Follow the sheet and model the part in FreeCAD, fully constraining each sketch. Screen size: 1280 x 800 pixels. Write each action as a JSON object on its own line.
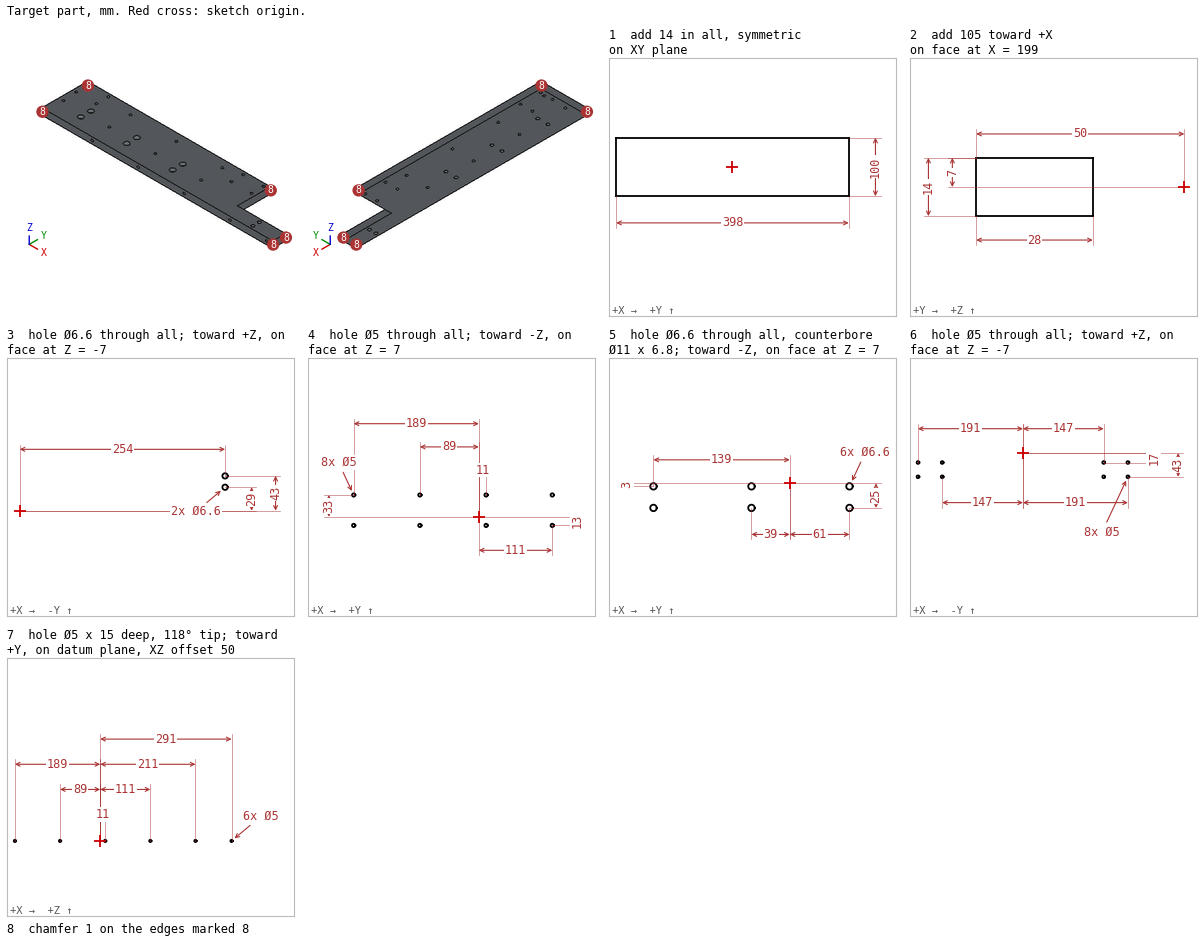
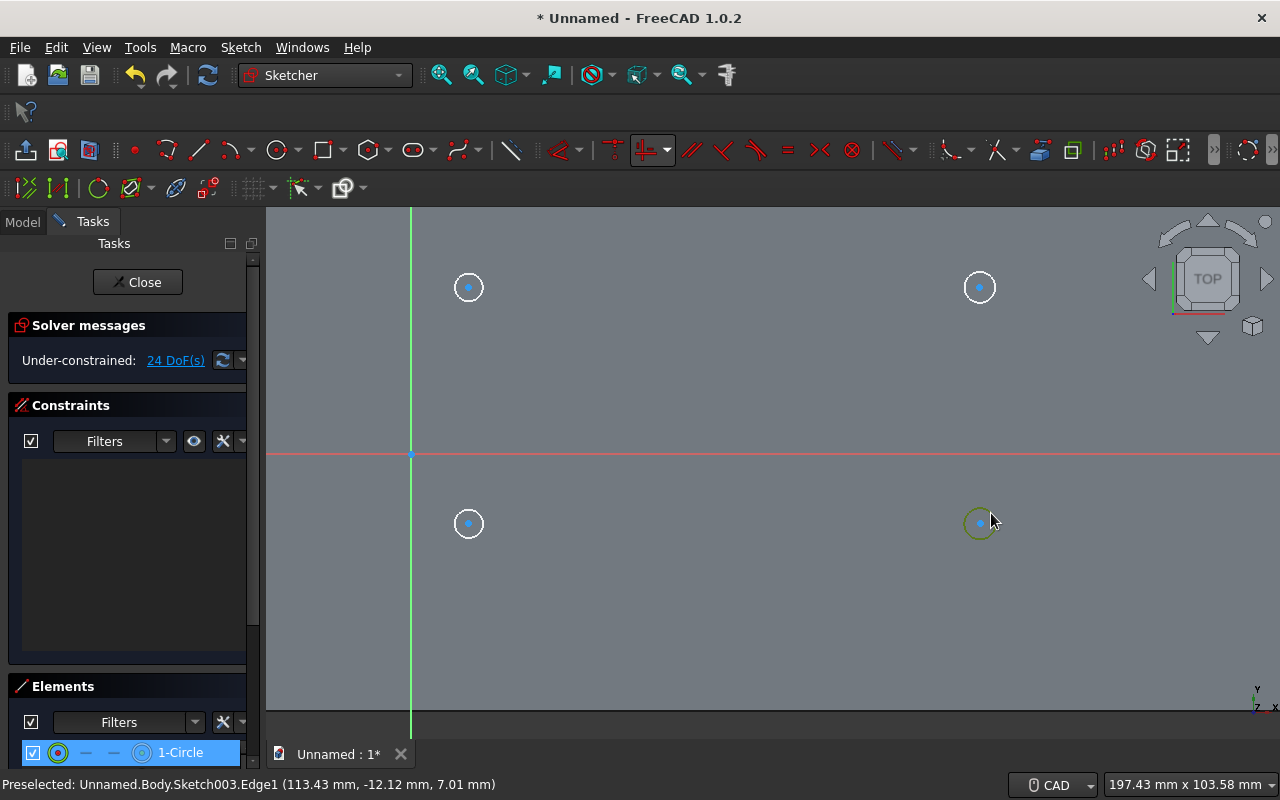
{"action": "scroll", "coordinate": [992, 514], "scroll_direction": "down", "scroll_amount": 5}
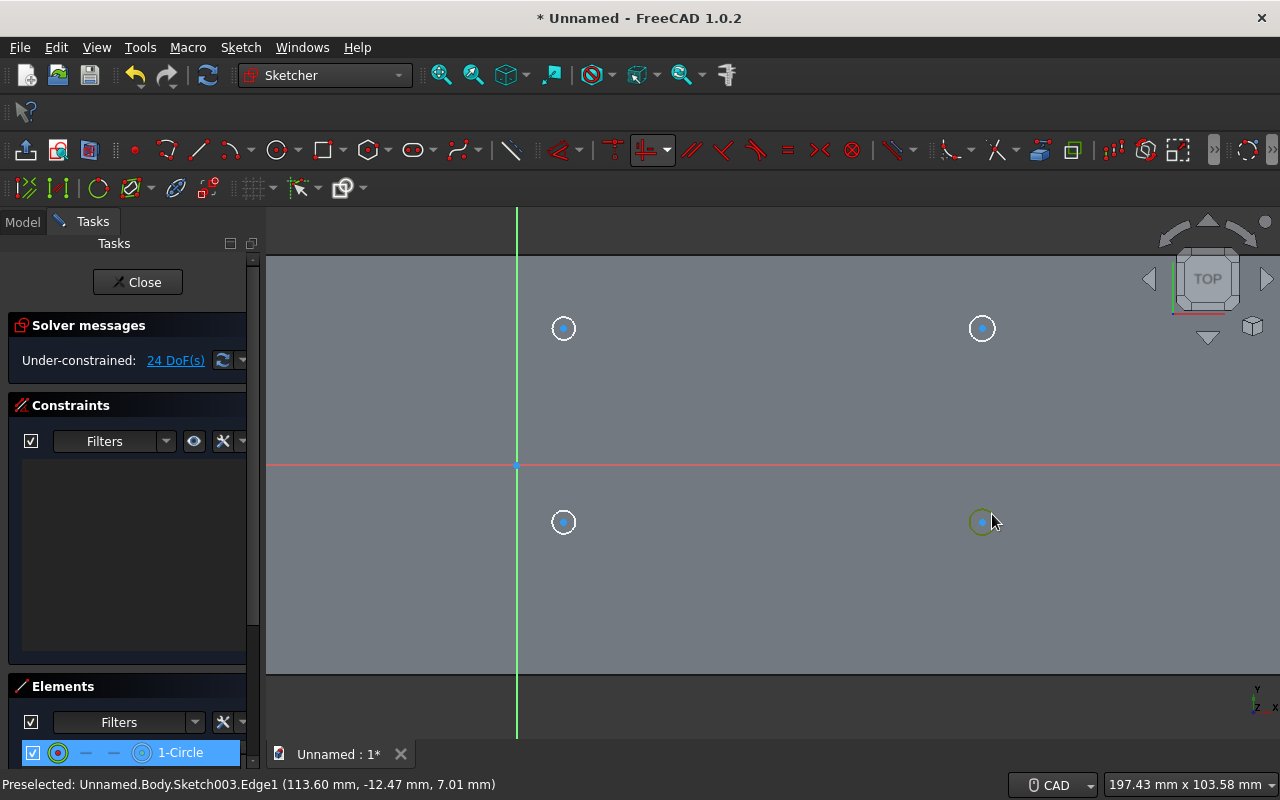
{"action": "scroll", "coordinate": [426, 427], "scroll_direction": "up", "scroll_amount": 6}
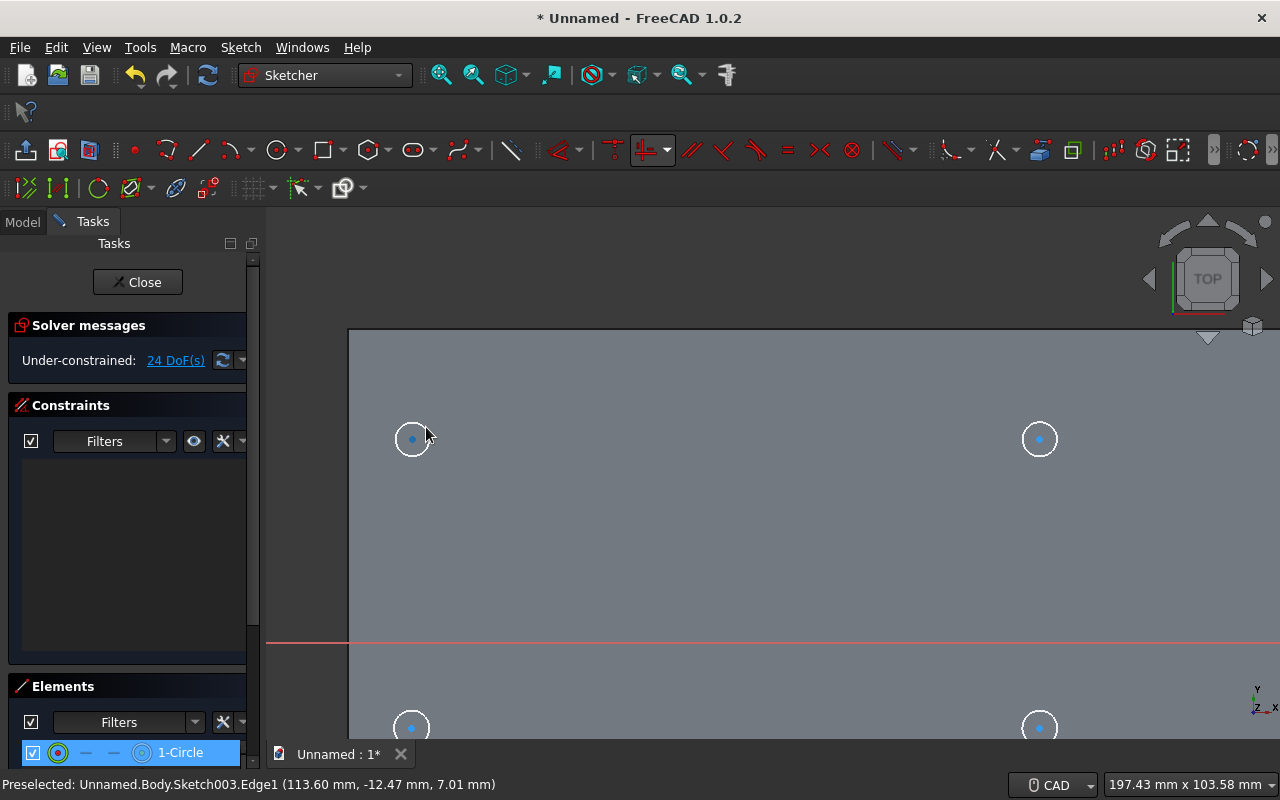
{"action": "left_click", "coordinate": [424, 427]}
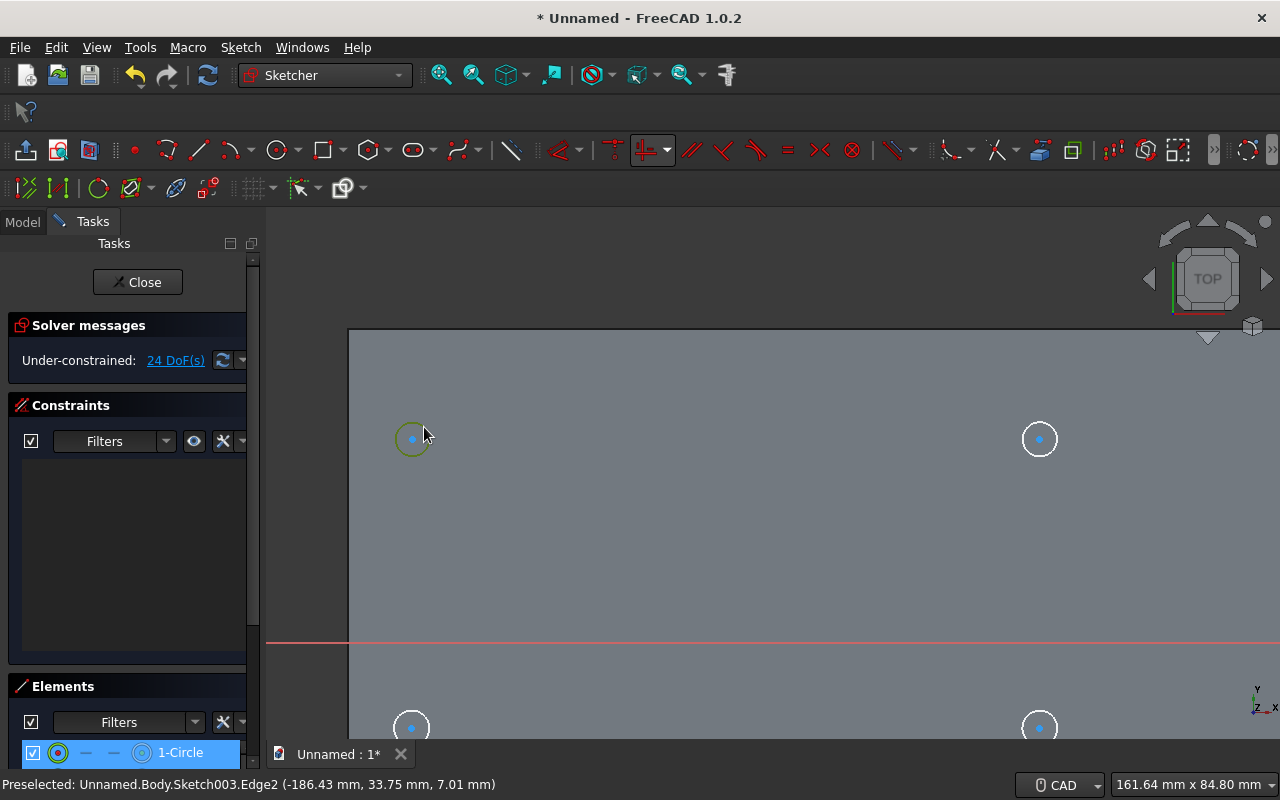
{"action": "left_click", "coordinate": [412, 711]}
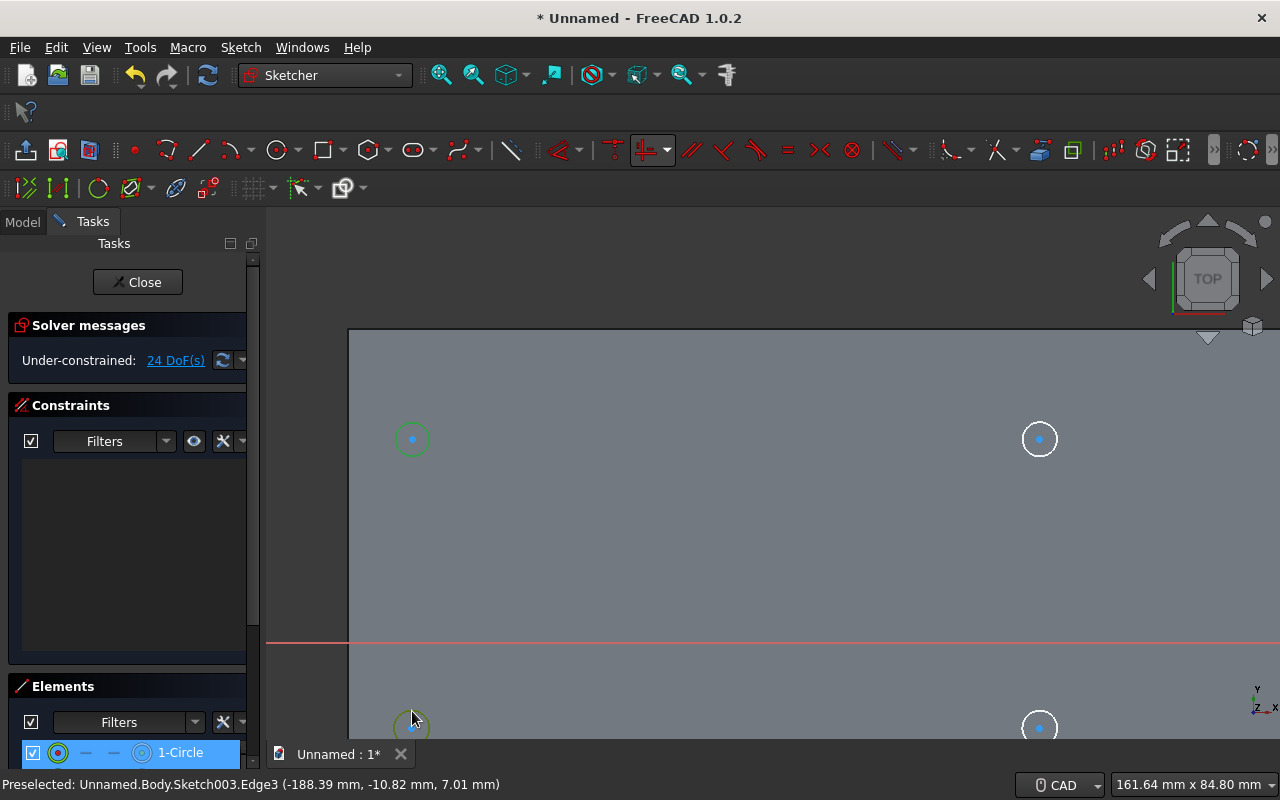
{"action": "left_click", "coordinate": [1052, 427]}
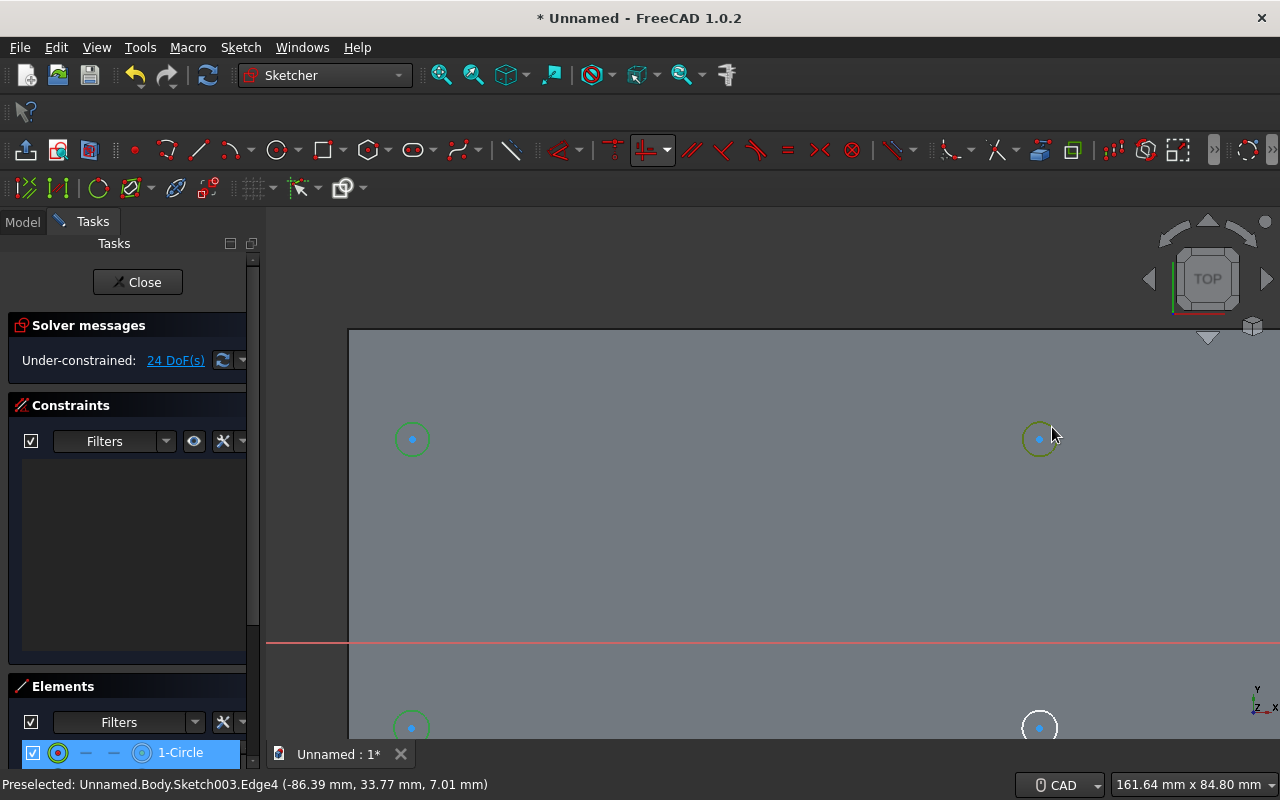
{"action": "left_click", "coordinate": [1040, 711]}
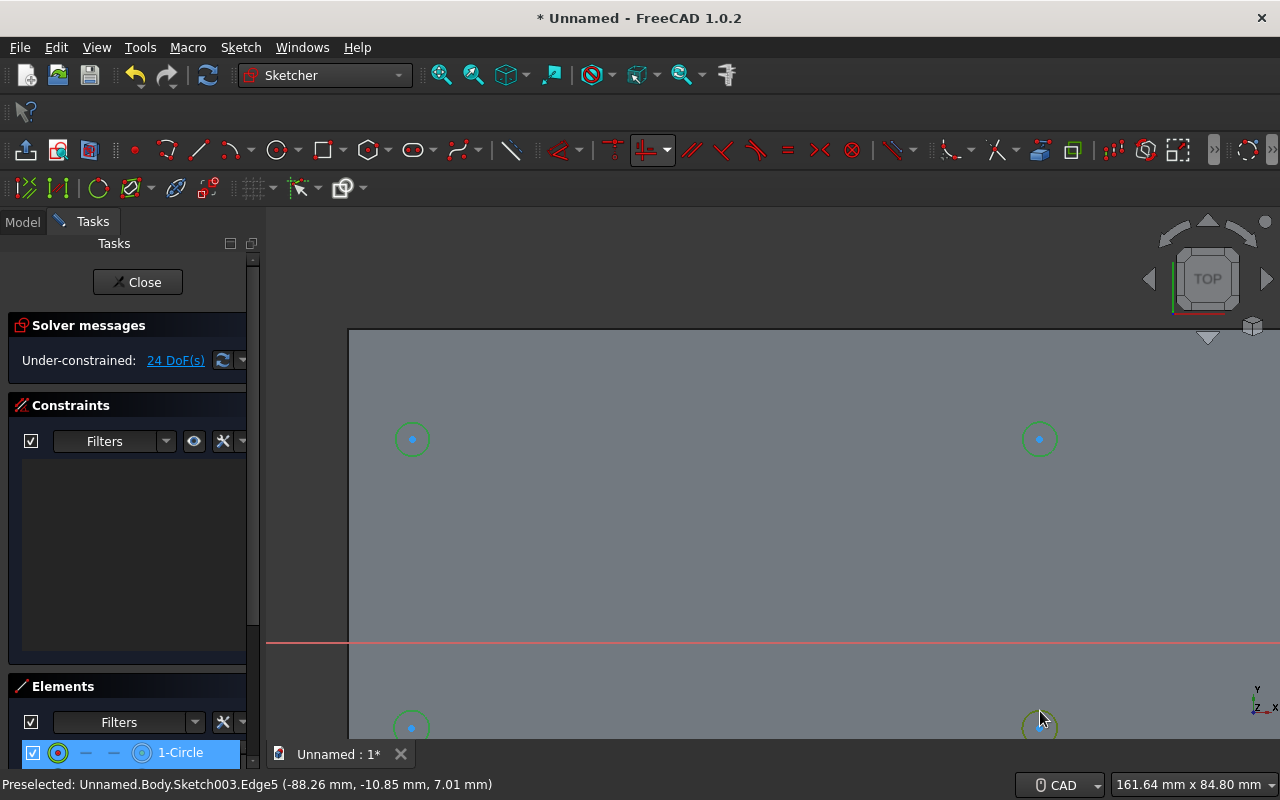
{"action": "scroll", "coordinate": [425, 427], "scroll_direction": "down", "scroll_amount": 6}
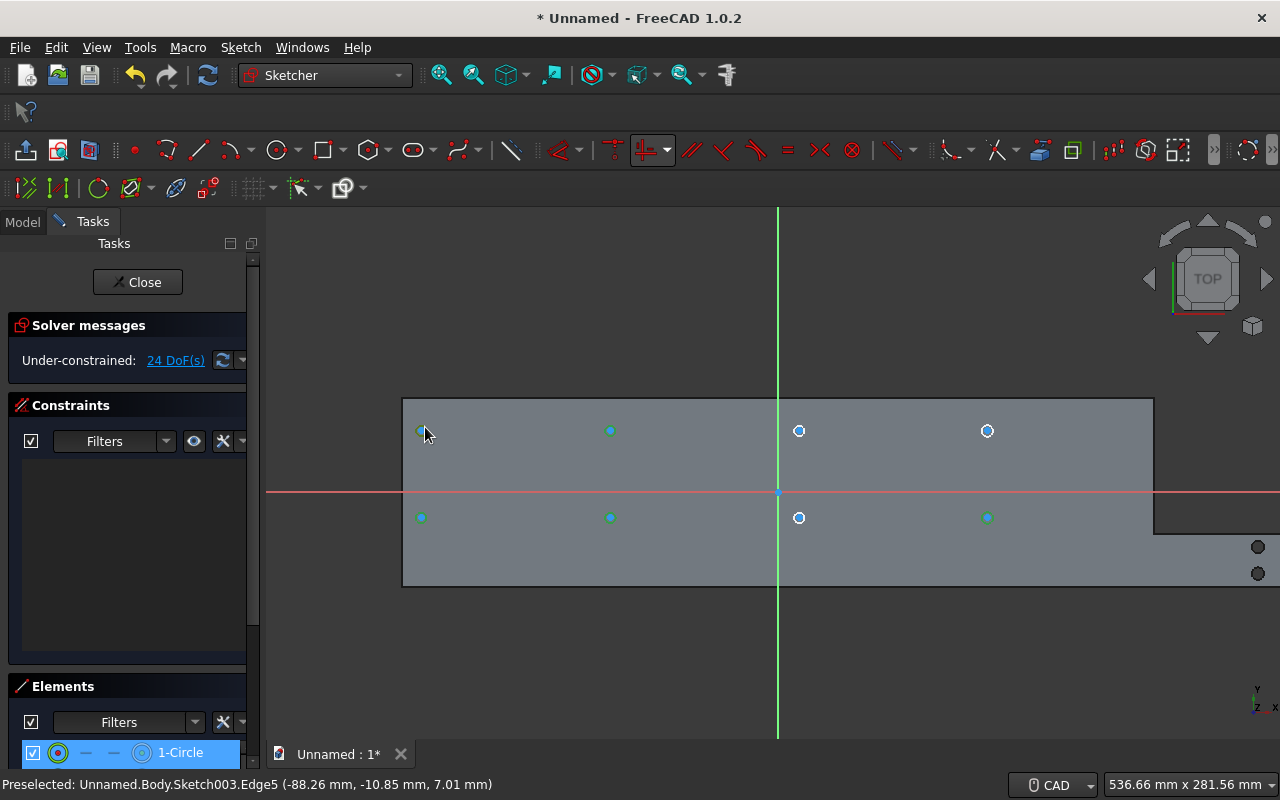
{"action": "scroll", "coordinate": [803, 427], "scroll_direction": "up", "scroll_amount": 5}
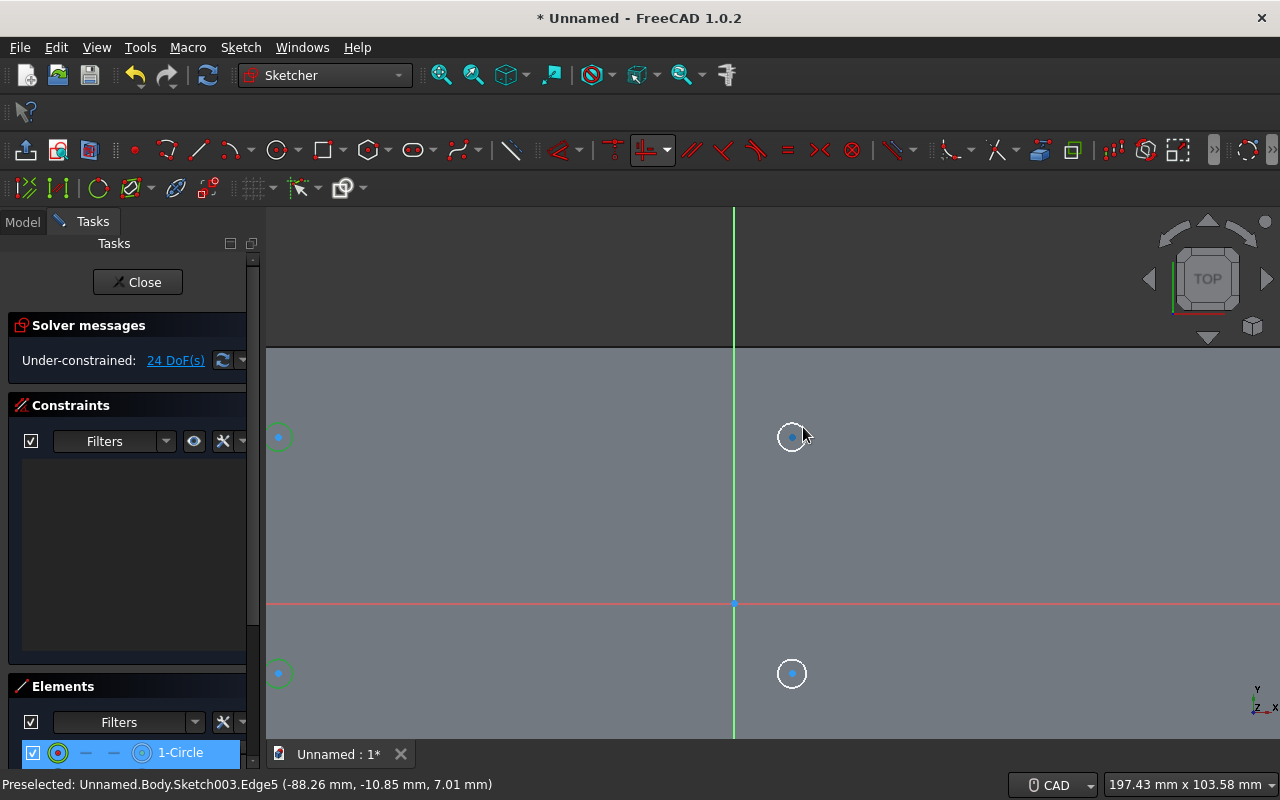
{"action": "left_click", "coordinate": [802, 427]}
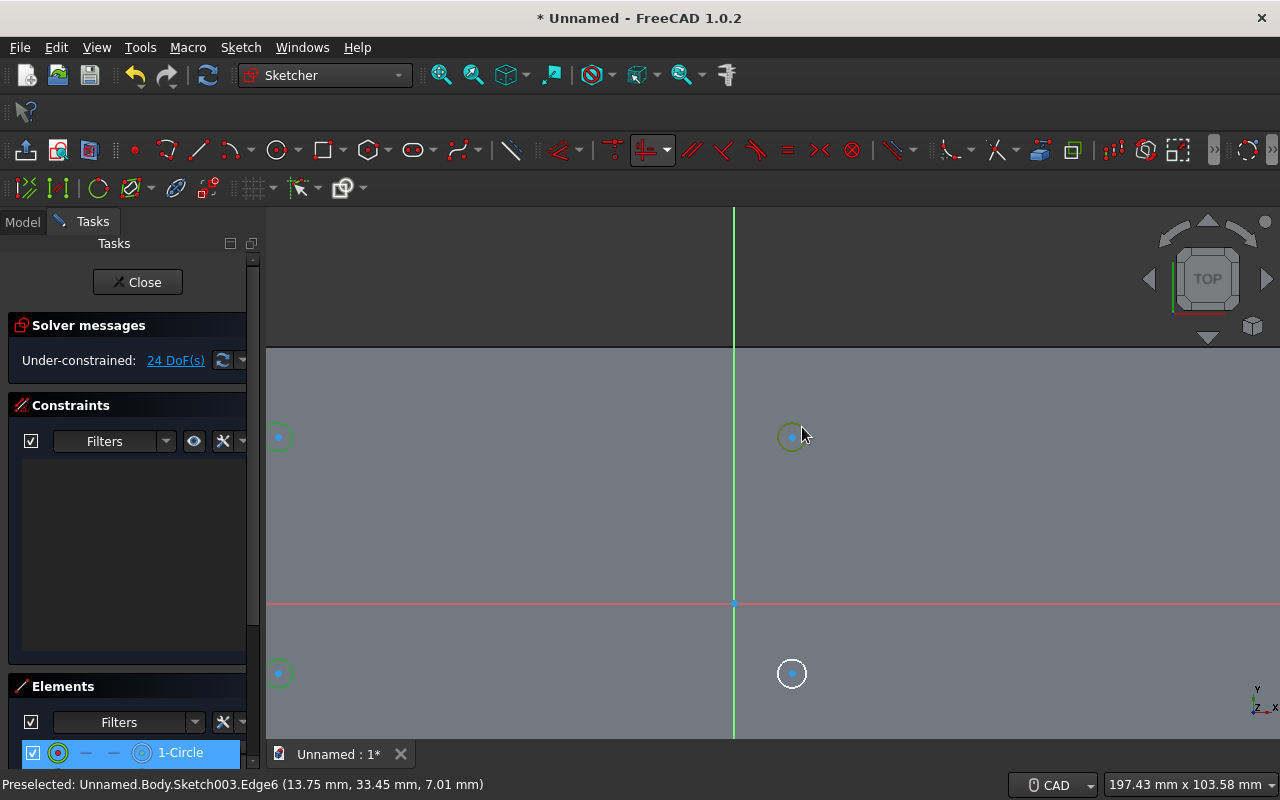
{"action": "left_click", "coordinate": [802, 664]}